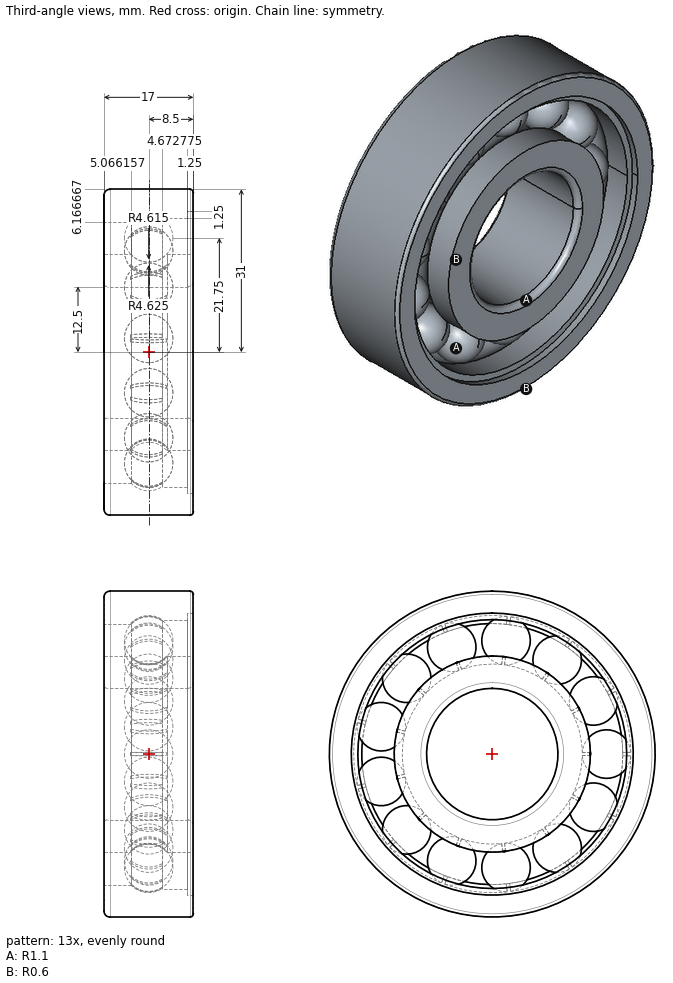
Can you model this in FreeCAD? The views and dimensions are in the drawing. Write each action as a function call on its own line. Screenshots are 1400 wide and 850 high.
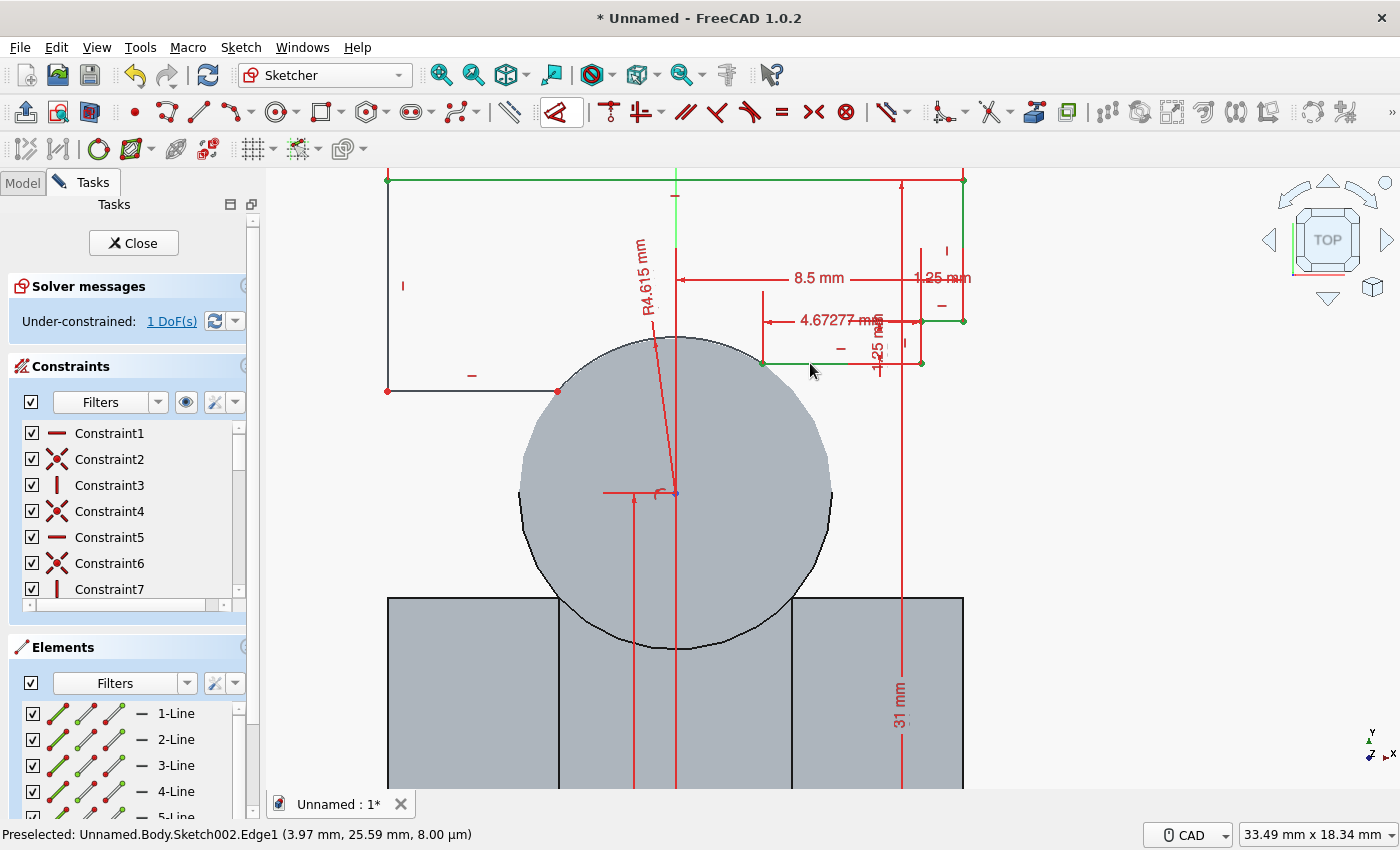
click(388, 244)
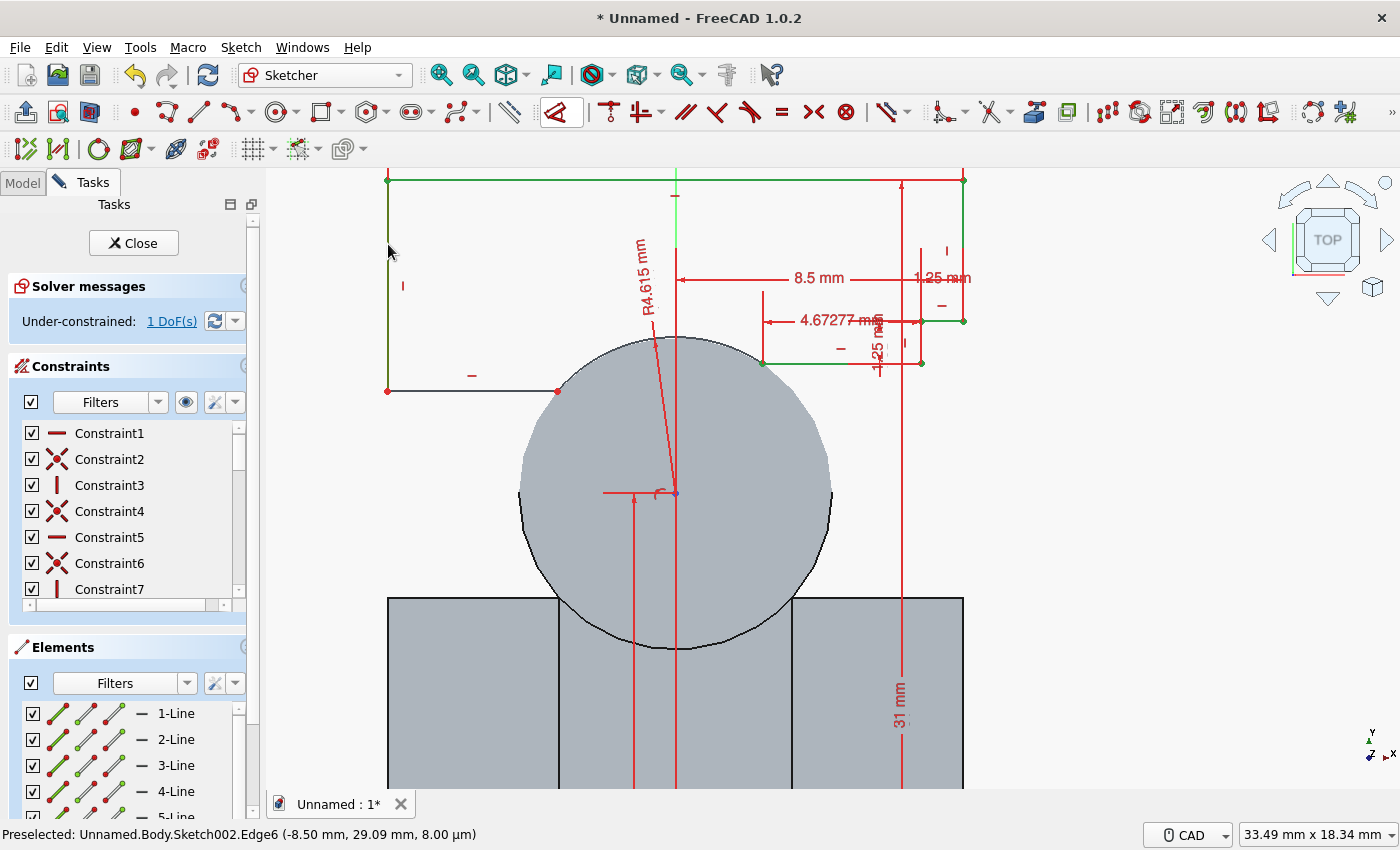
key(i)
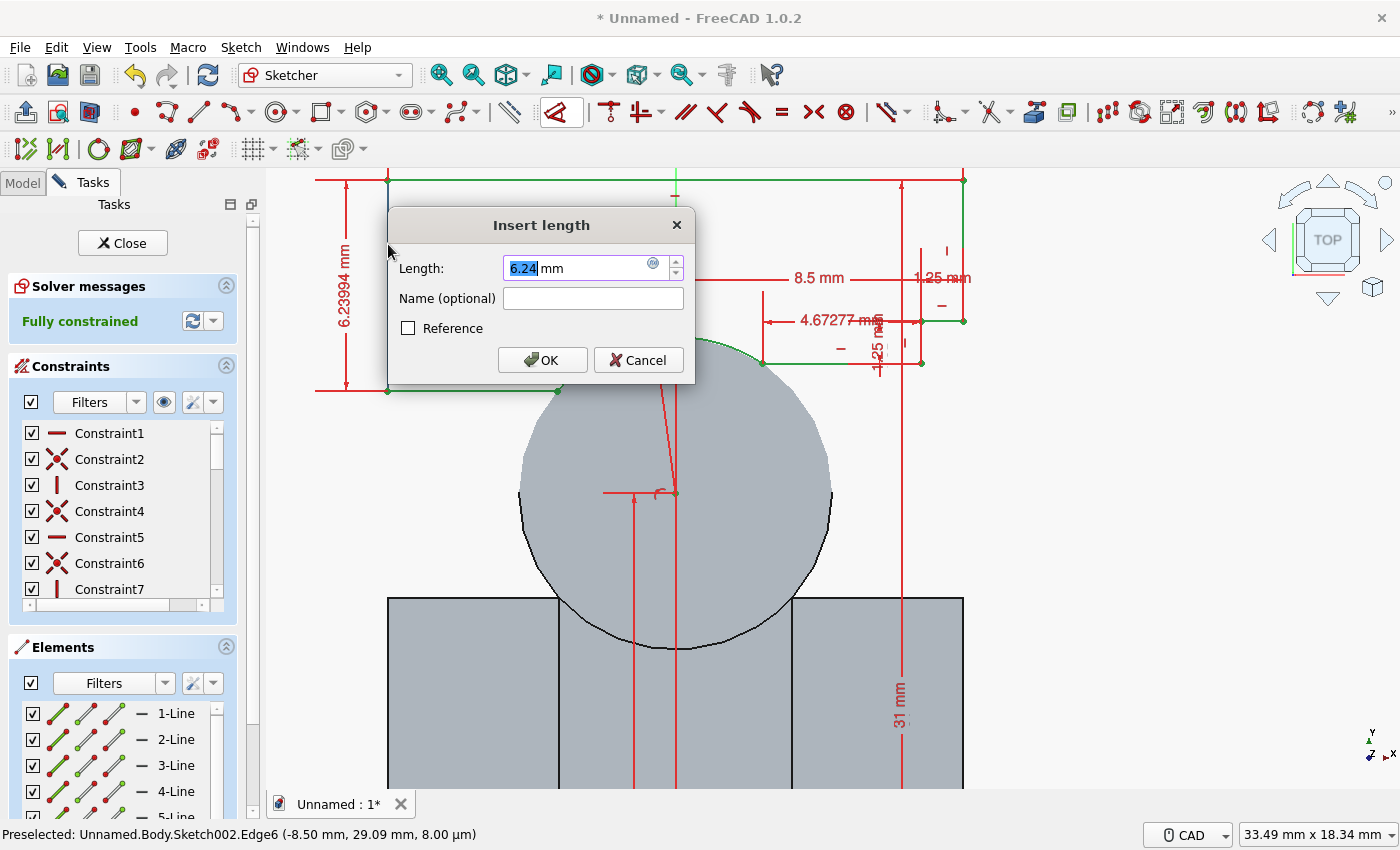
text(6.166667)
key(Return)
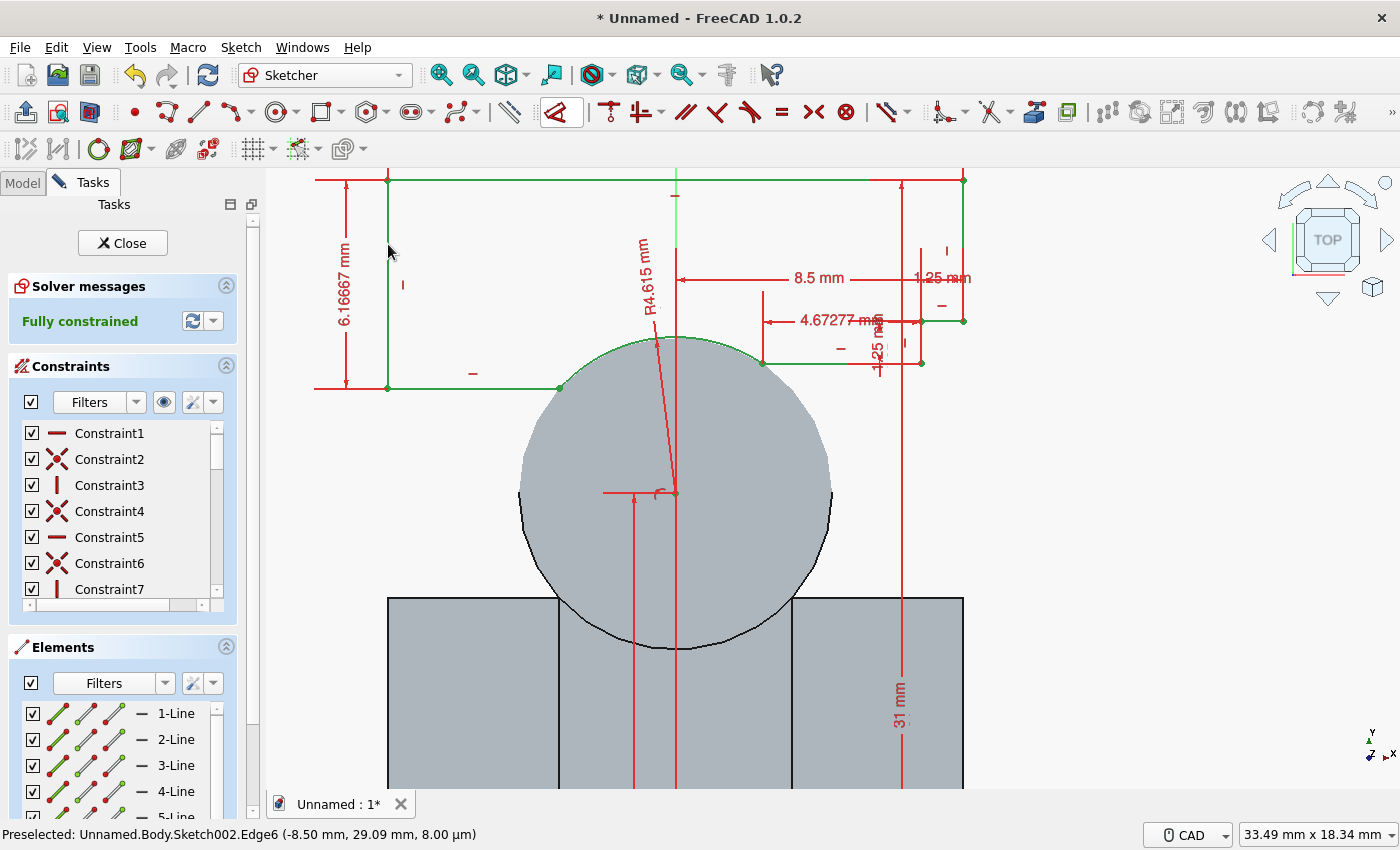
click(123, 243)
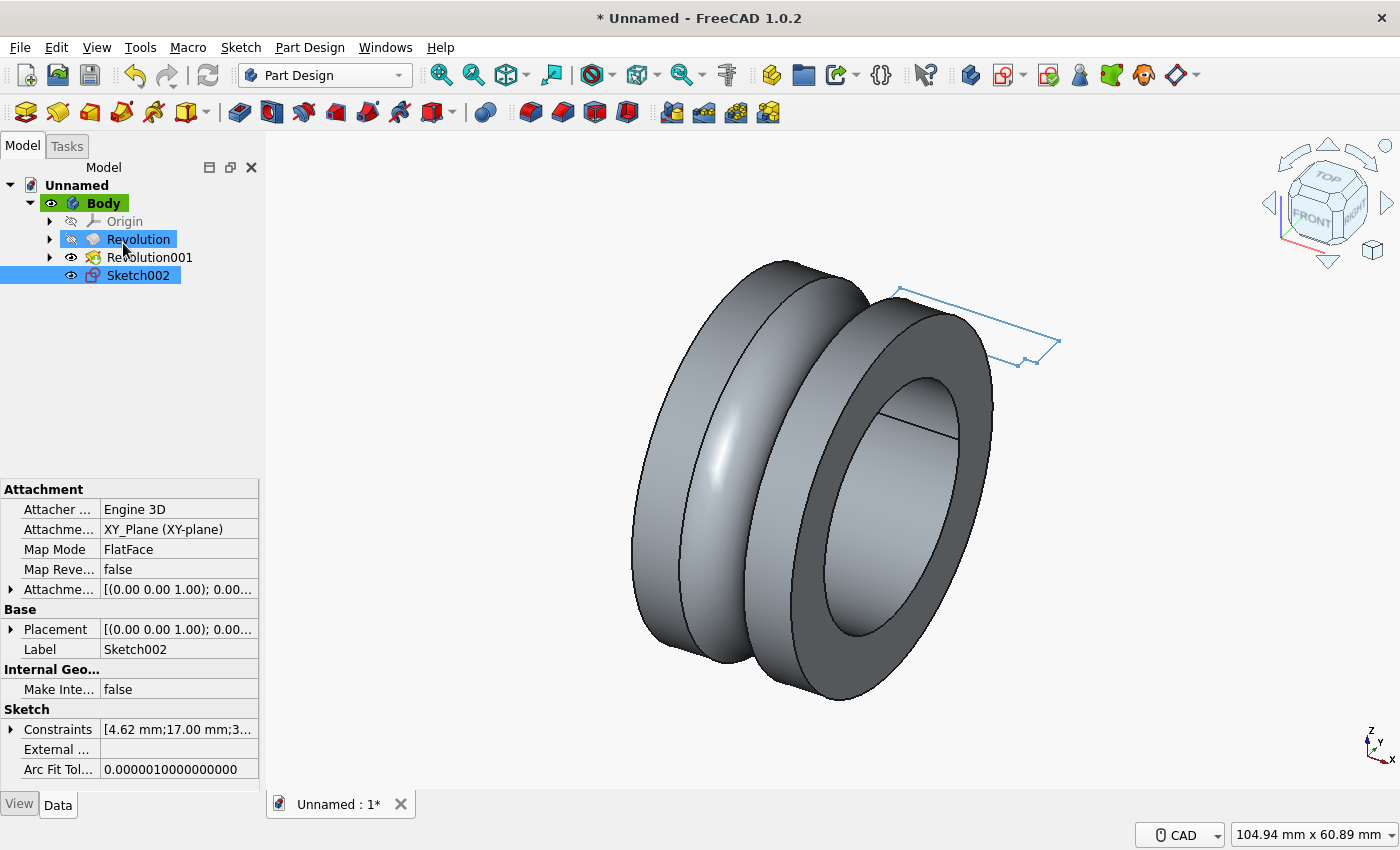
click(58, 112)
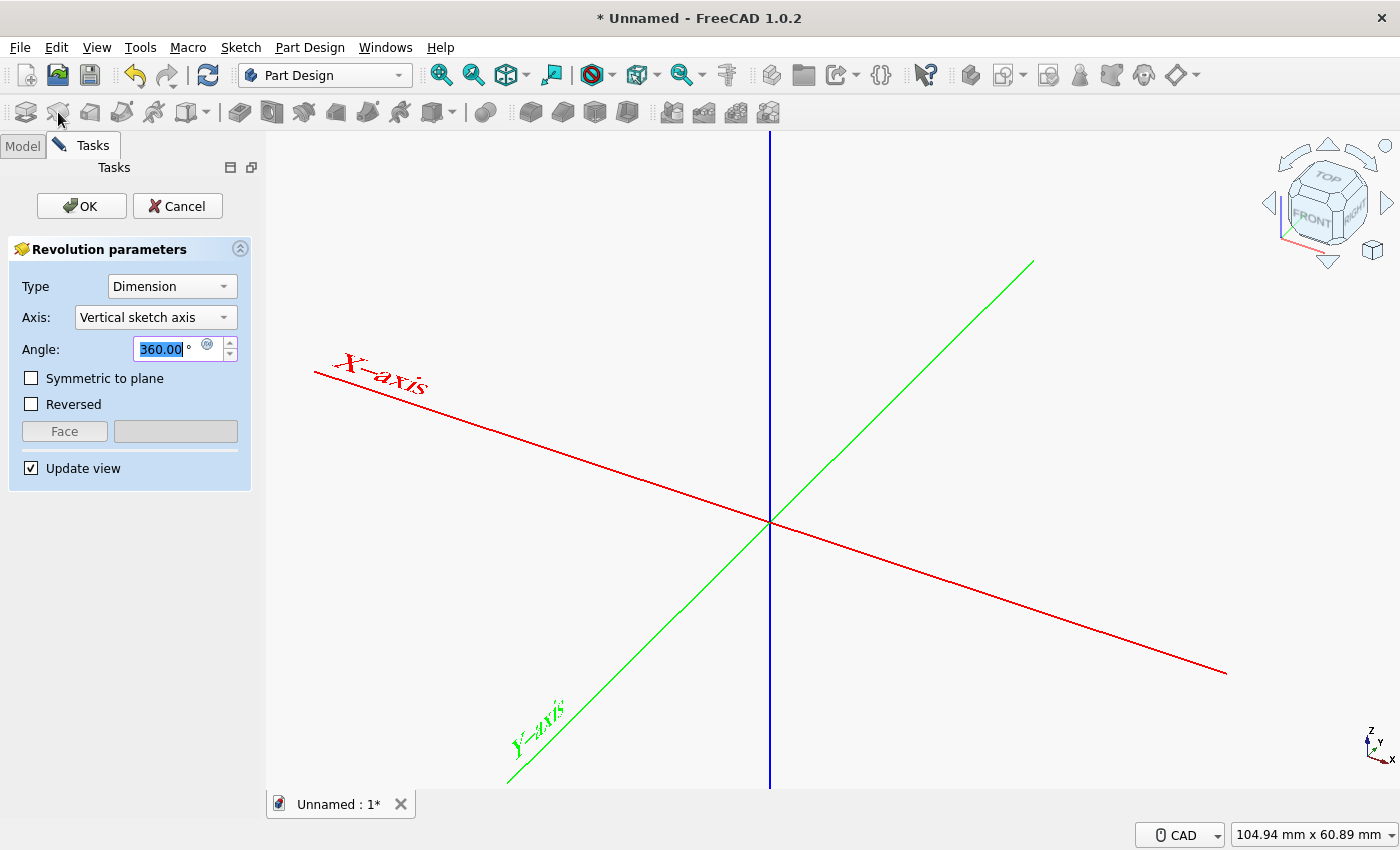
click(156, 318)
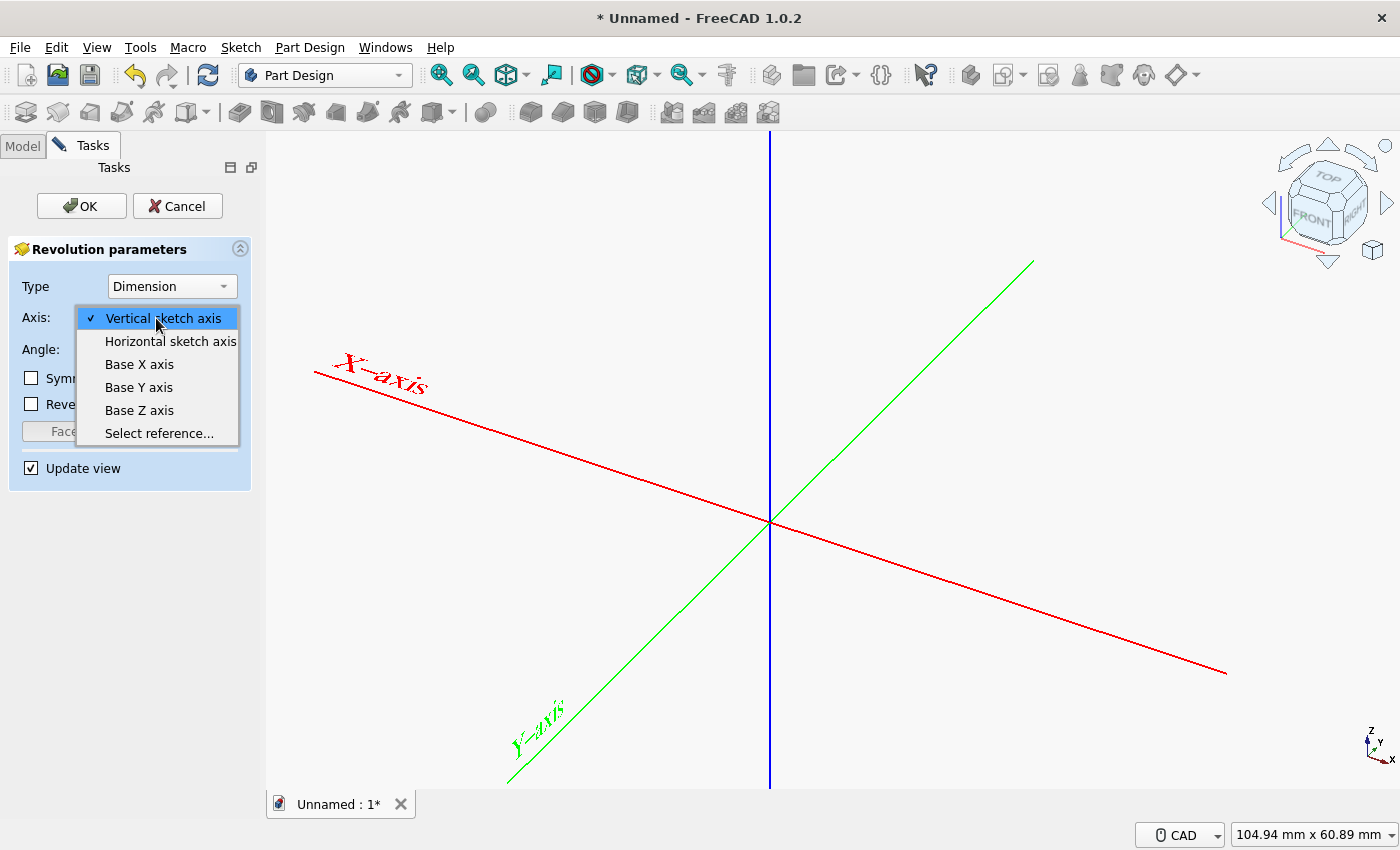
click(156, 342)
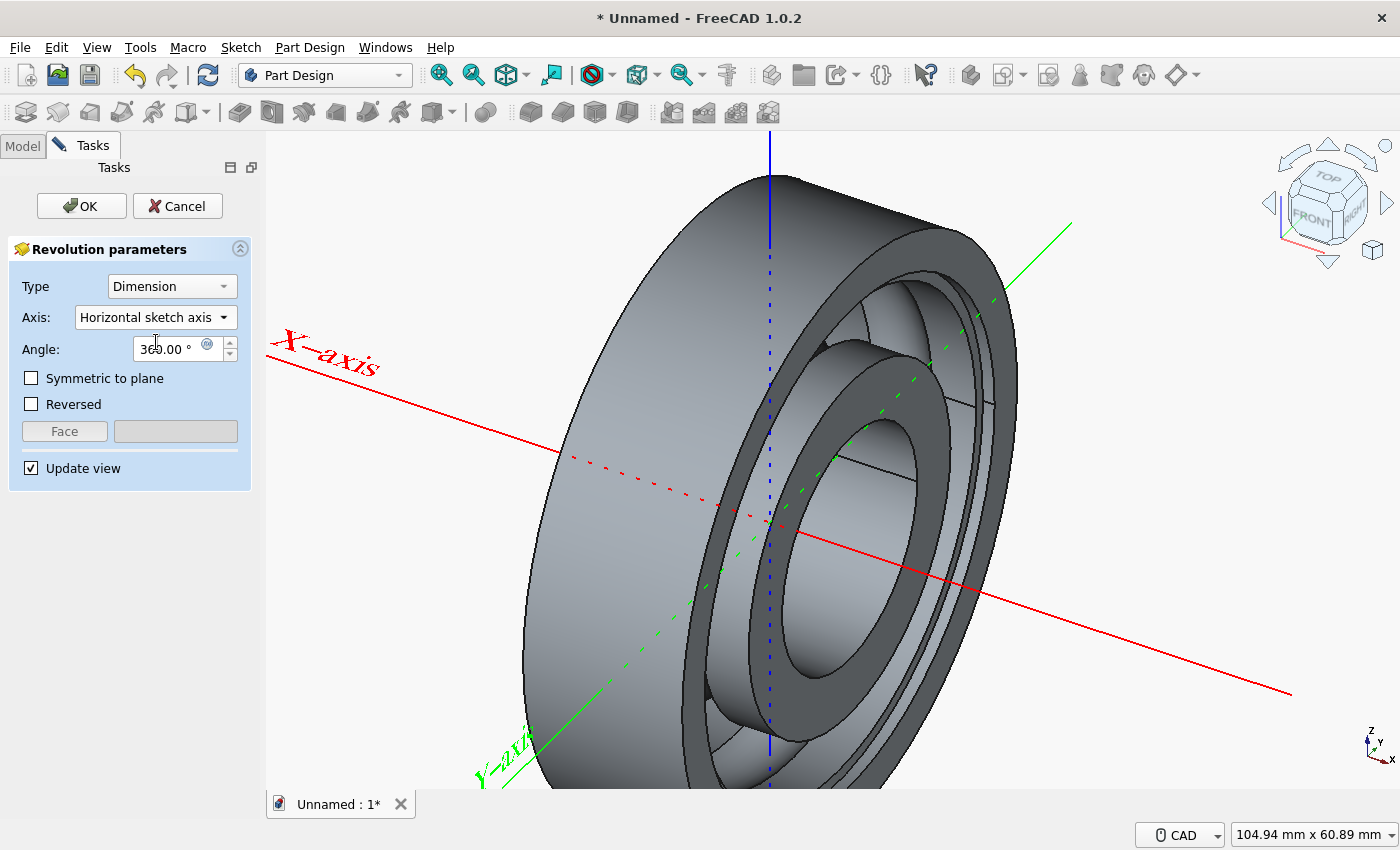
click(82, 206)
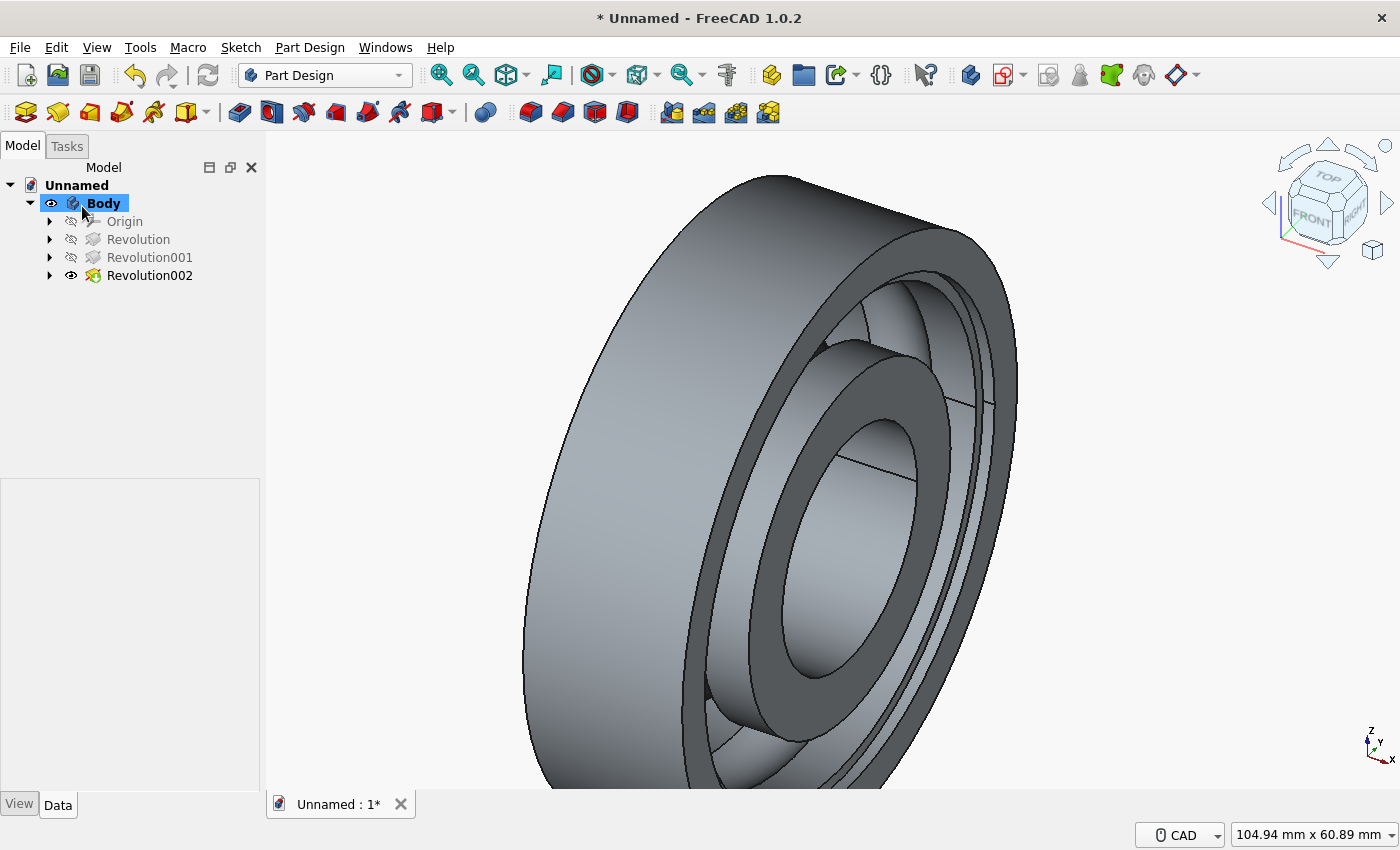
click(442, 76)